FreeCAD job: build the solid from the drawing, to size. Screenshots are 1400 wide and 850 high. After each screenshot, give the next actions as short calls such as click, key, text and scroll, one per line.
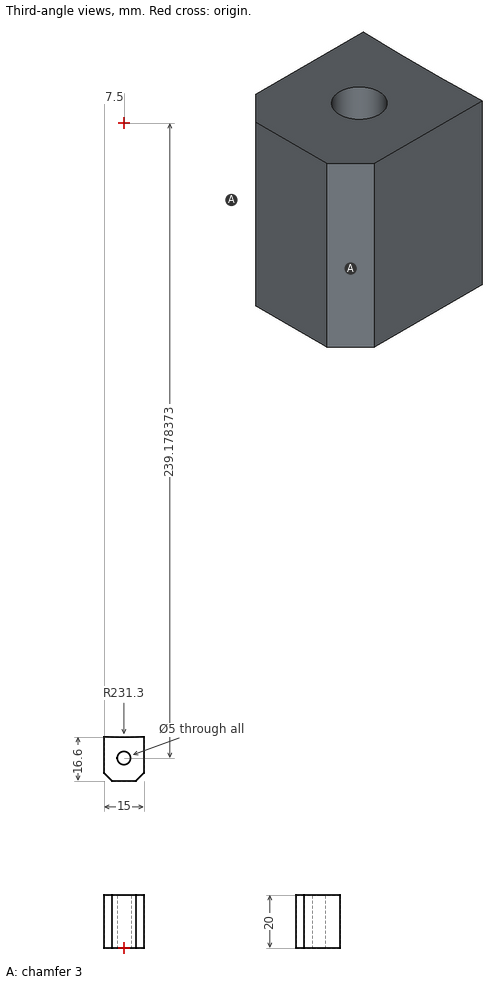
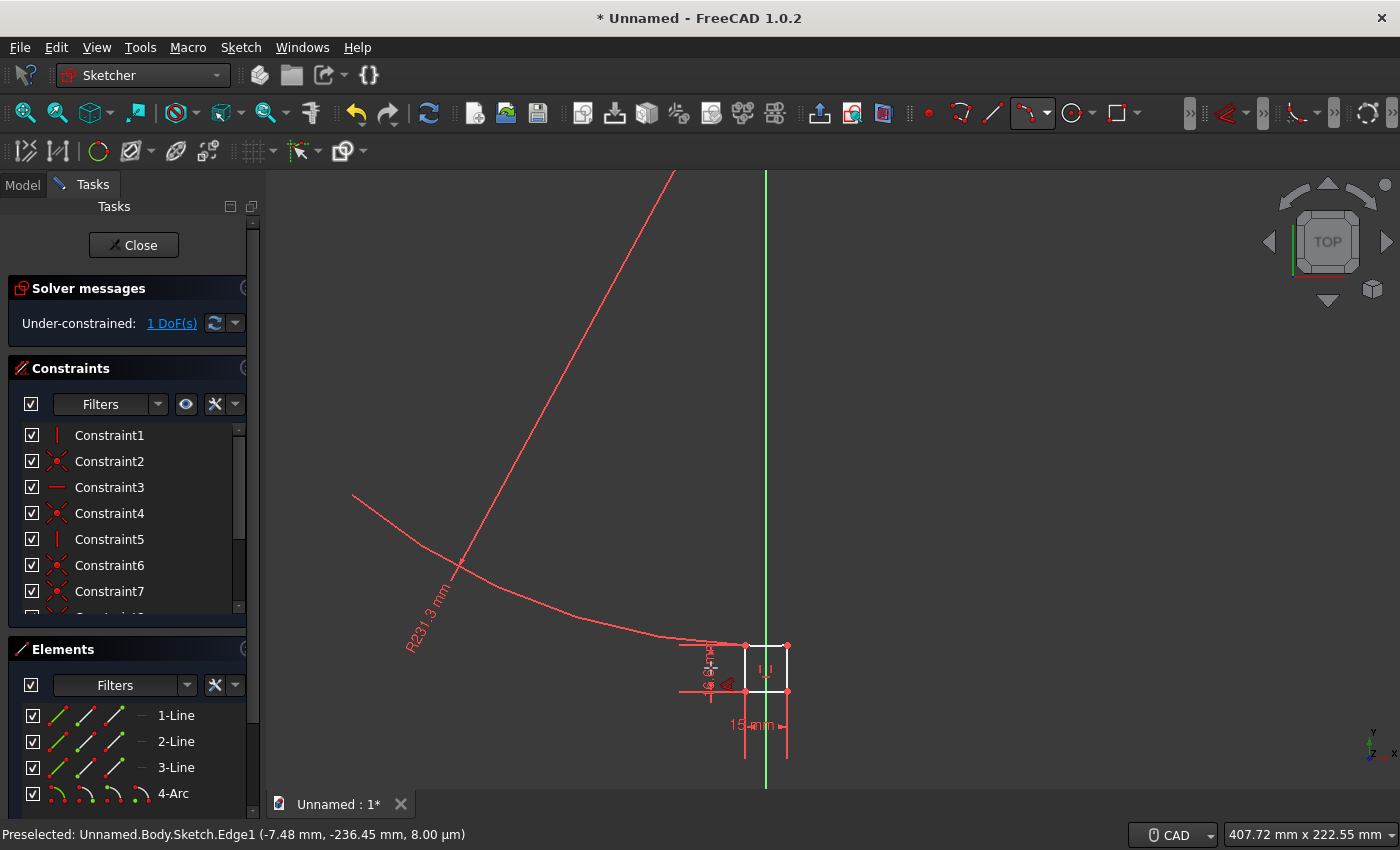
scroll(745, 645, up, 4)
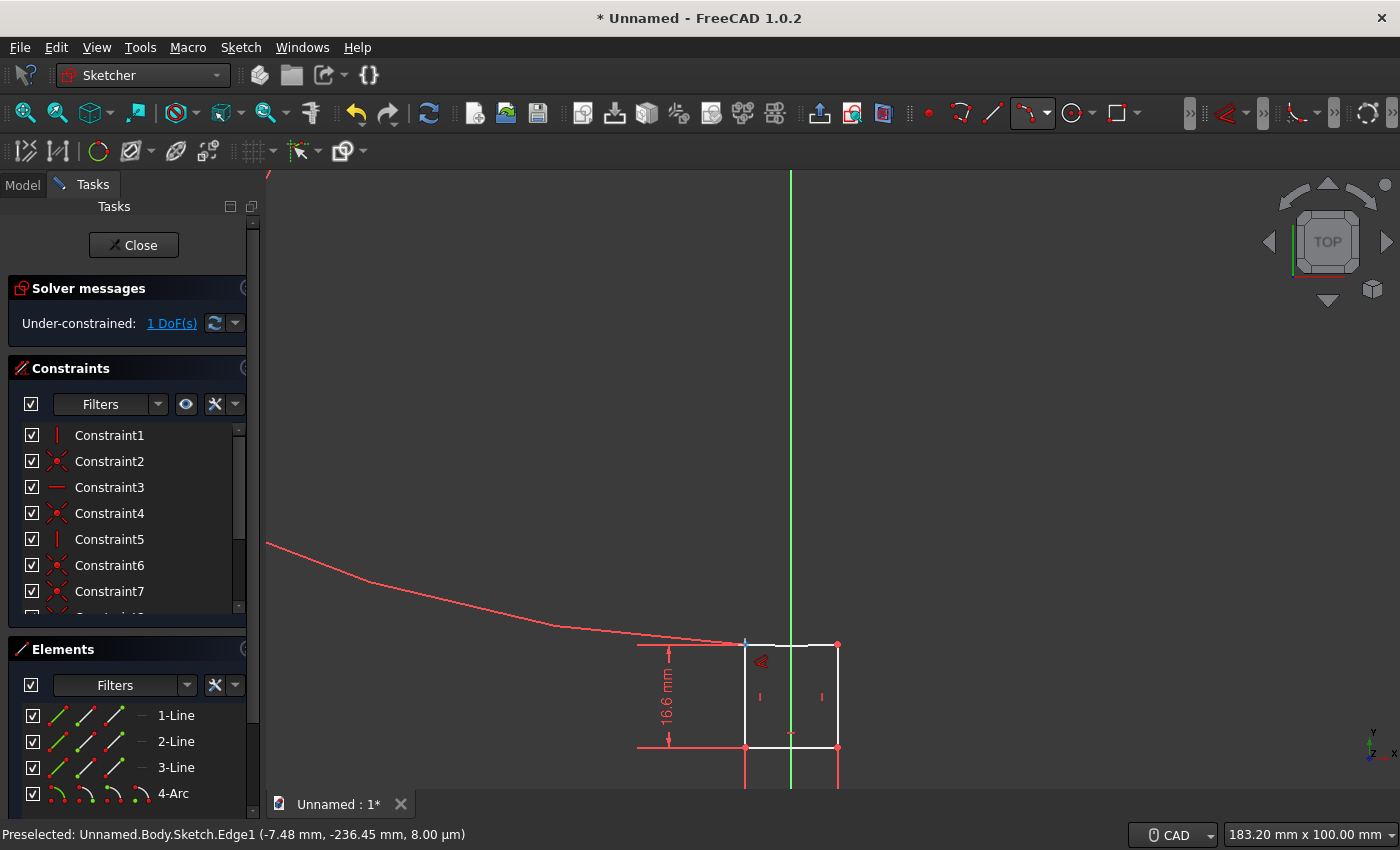
click(745, 645)
click(768, 679)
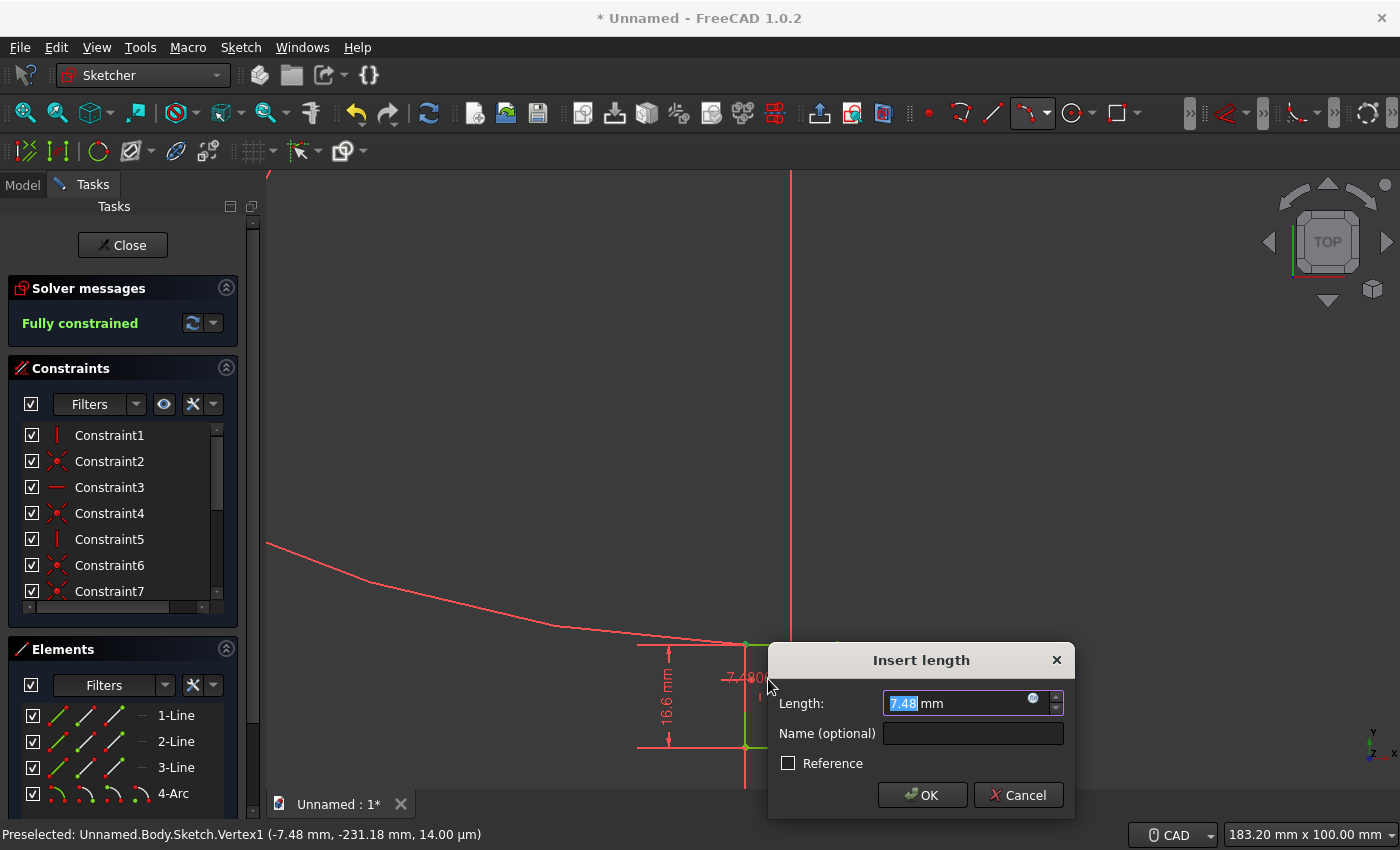
text(7.5)
key(Return)
key(Escape)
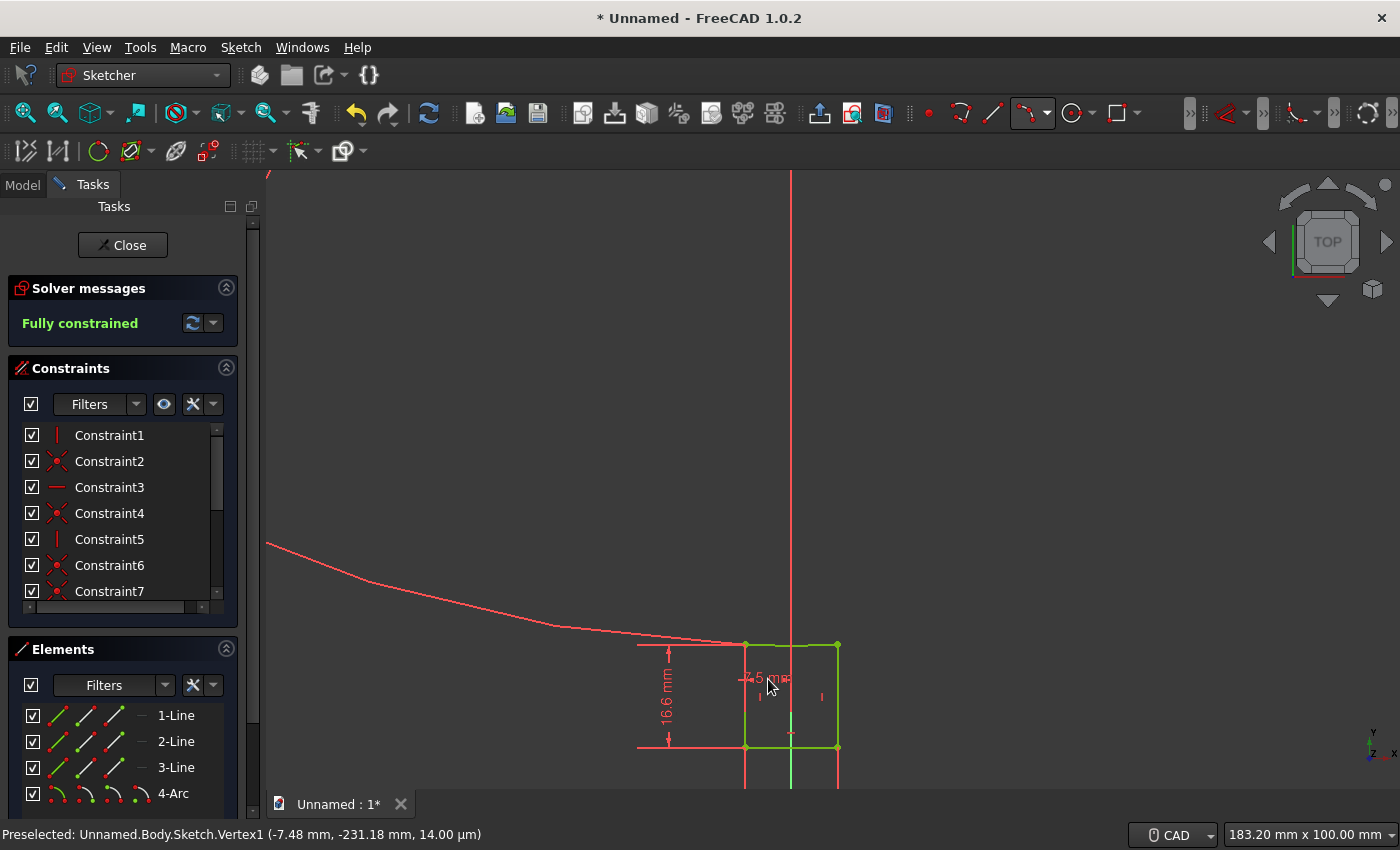
click(123, 245)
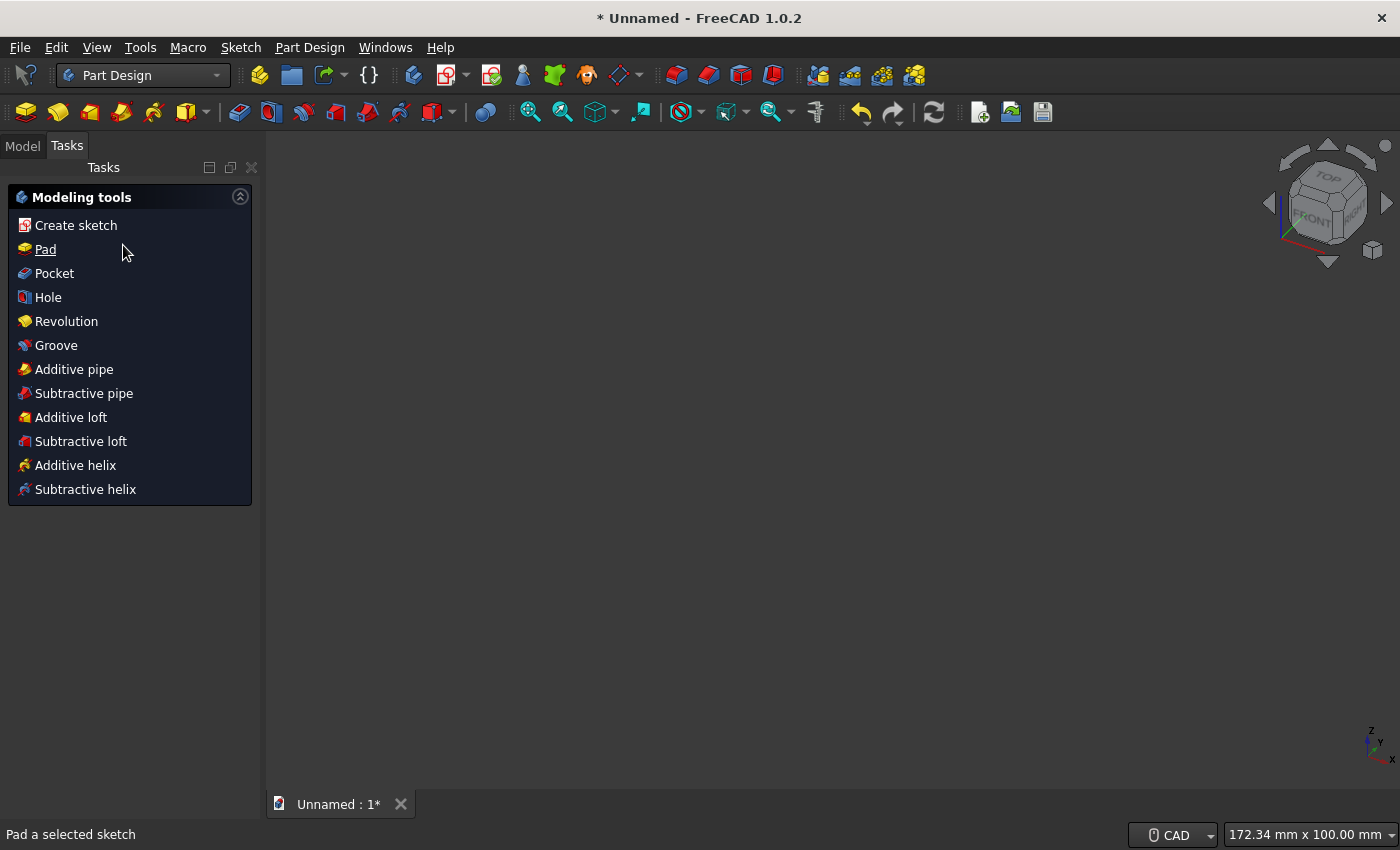
click(26, 112)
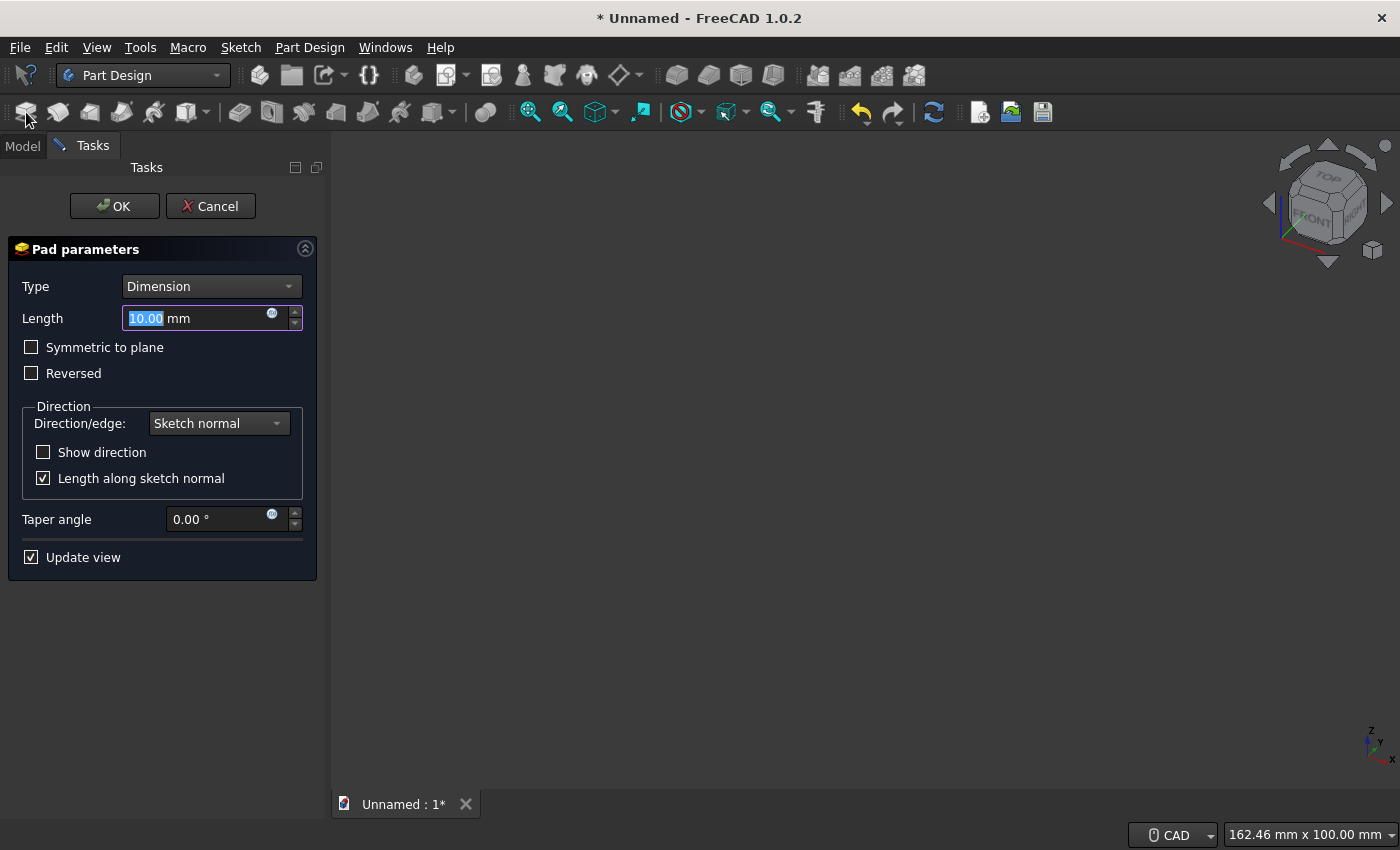
text(20)
key(Tab)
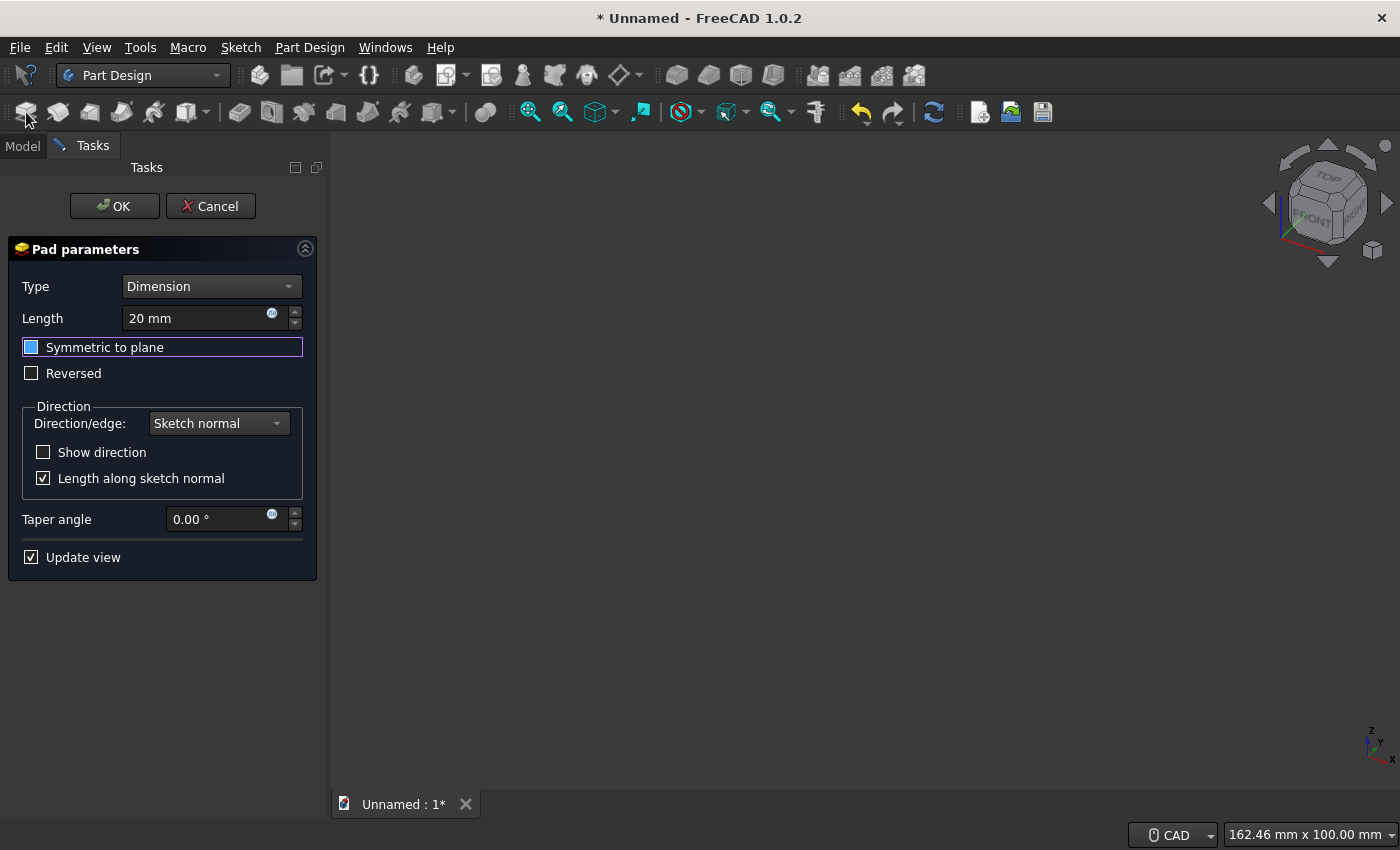
click(115, 206)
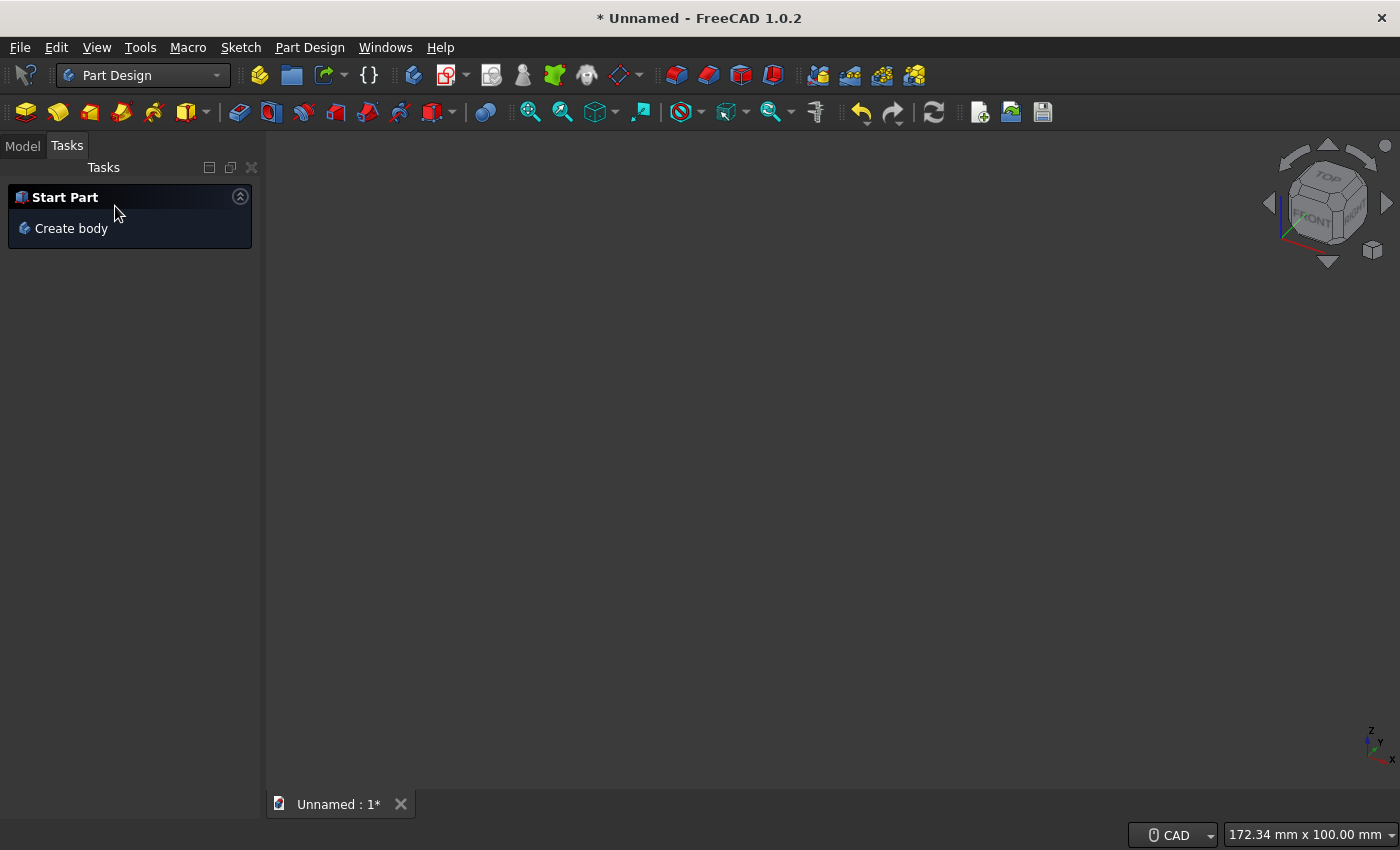
click(532, 112)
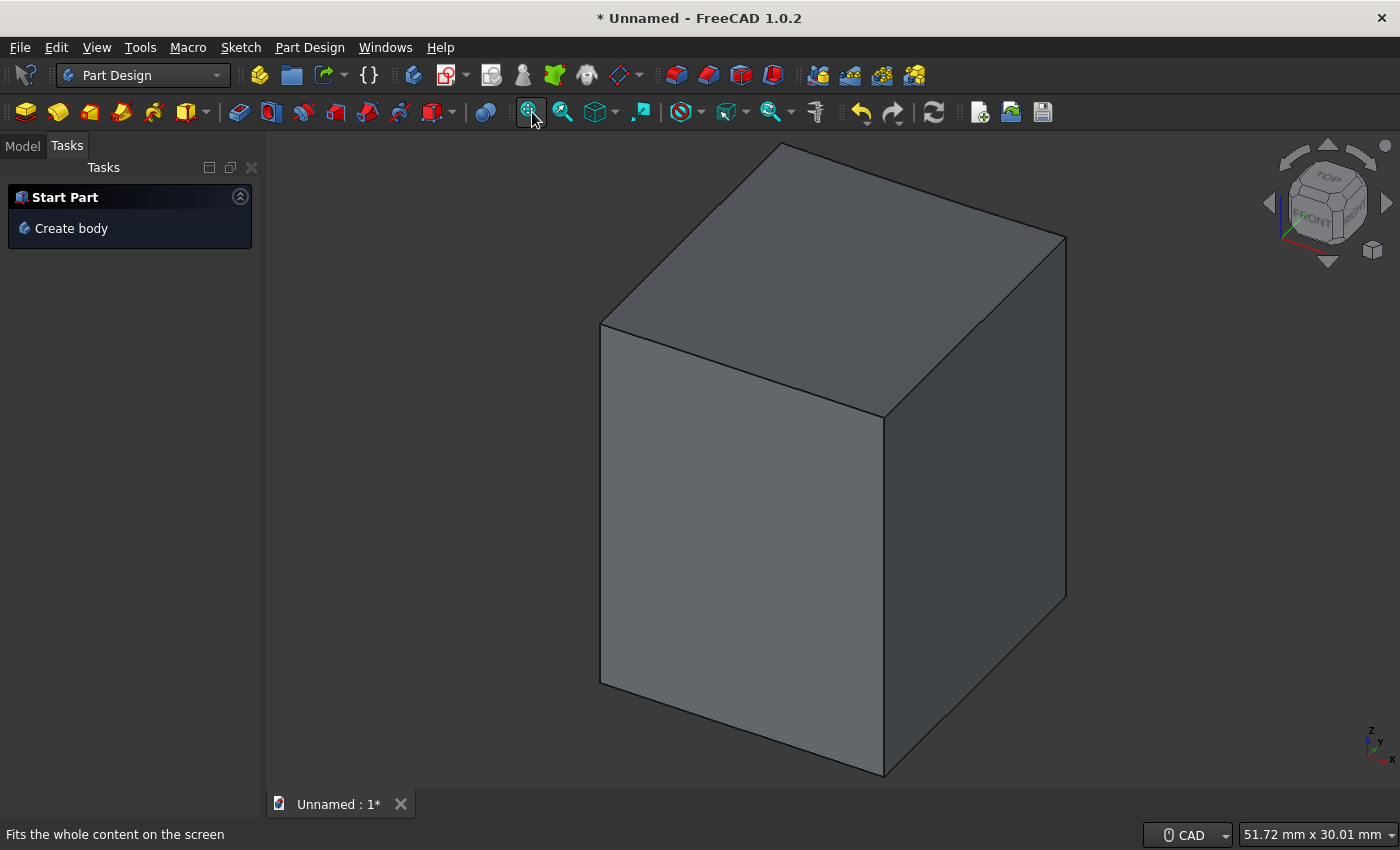
click(884, 597)